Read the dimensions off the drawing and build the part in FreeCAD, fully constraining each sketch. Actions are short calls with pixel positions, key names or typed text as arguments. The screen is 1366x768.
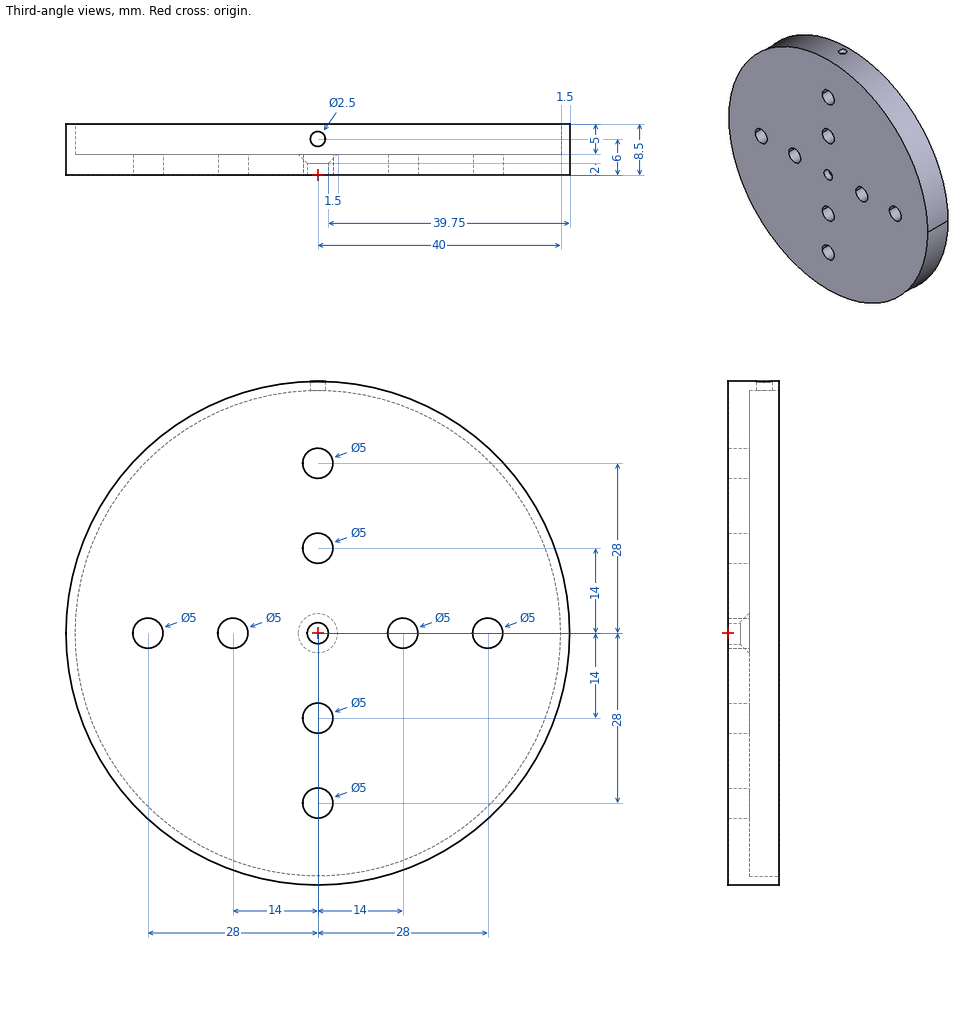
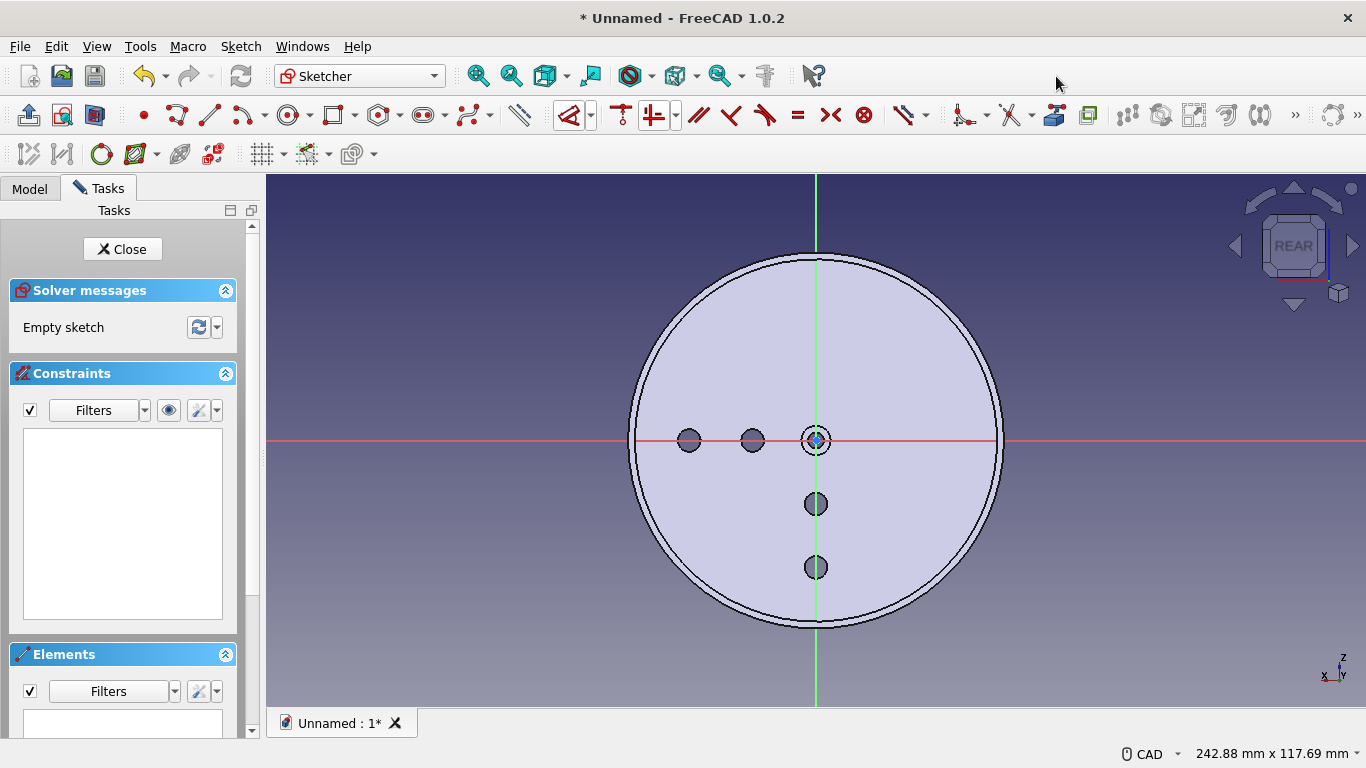
scroll(821, 372, up, 13)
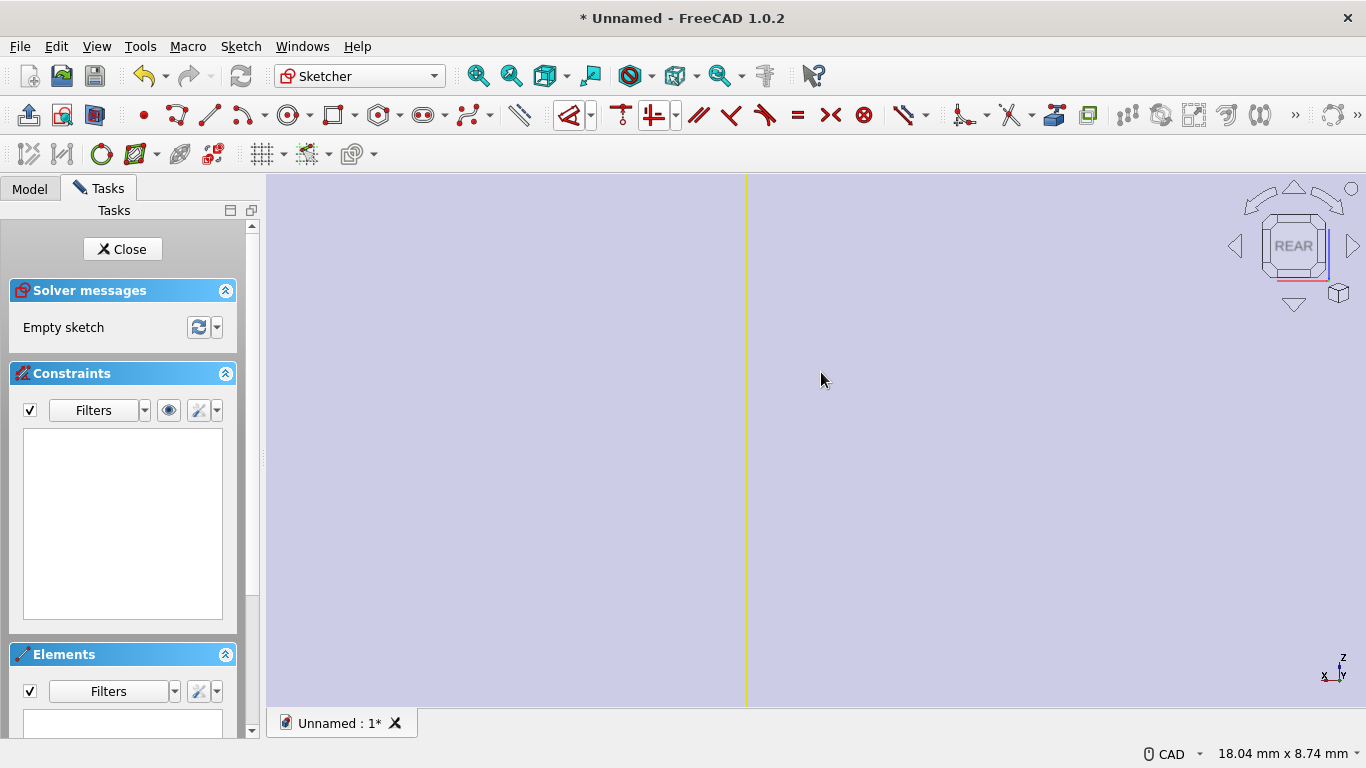
click(288, 116)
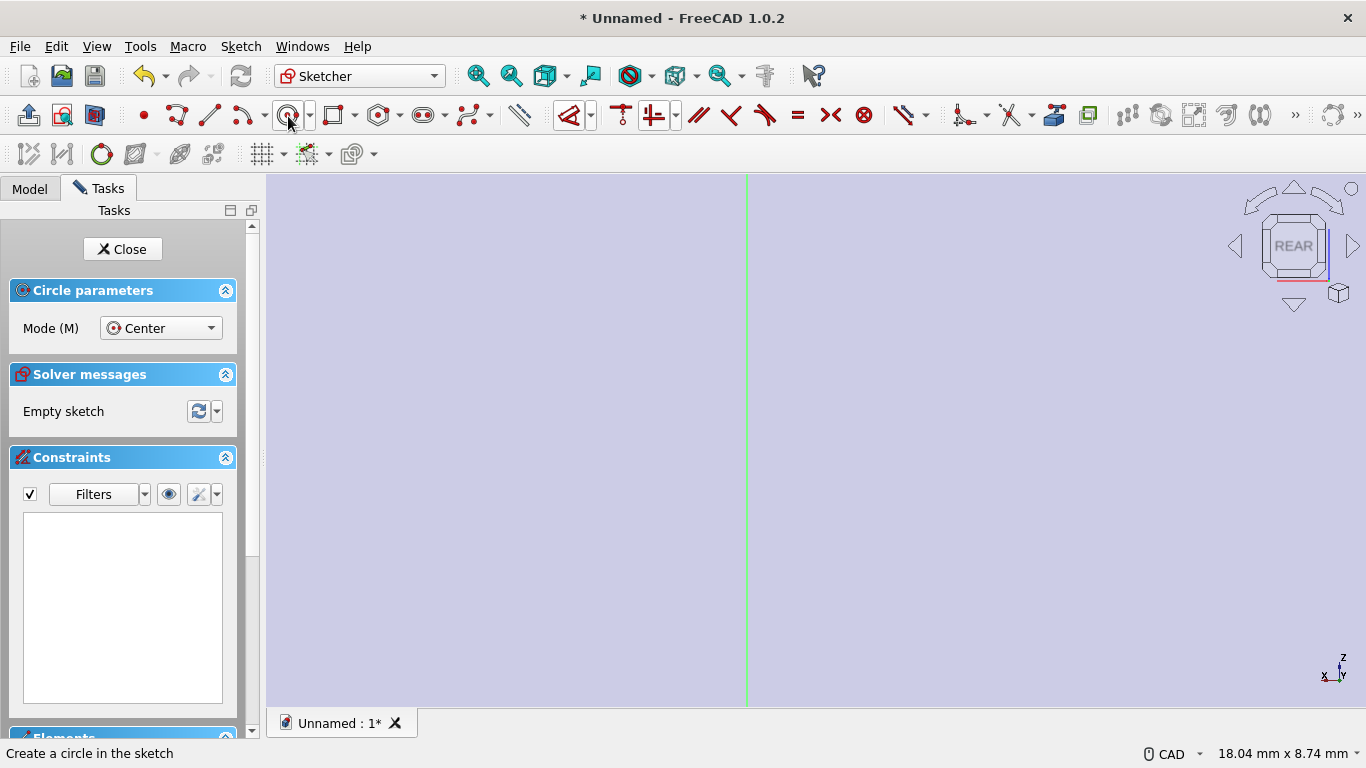
click(747, 436)
click(855, 328)
key(Escape)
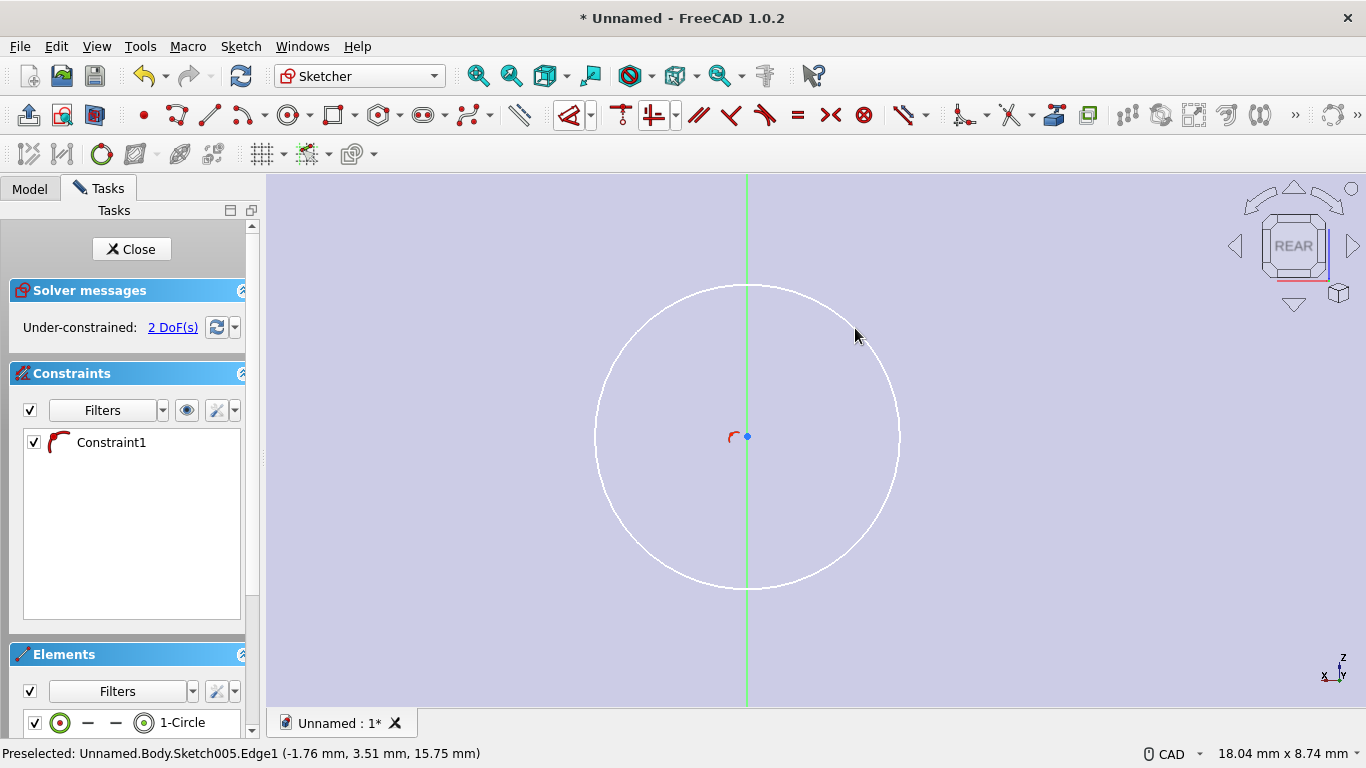
click(855, 329)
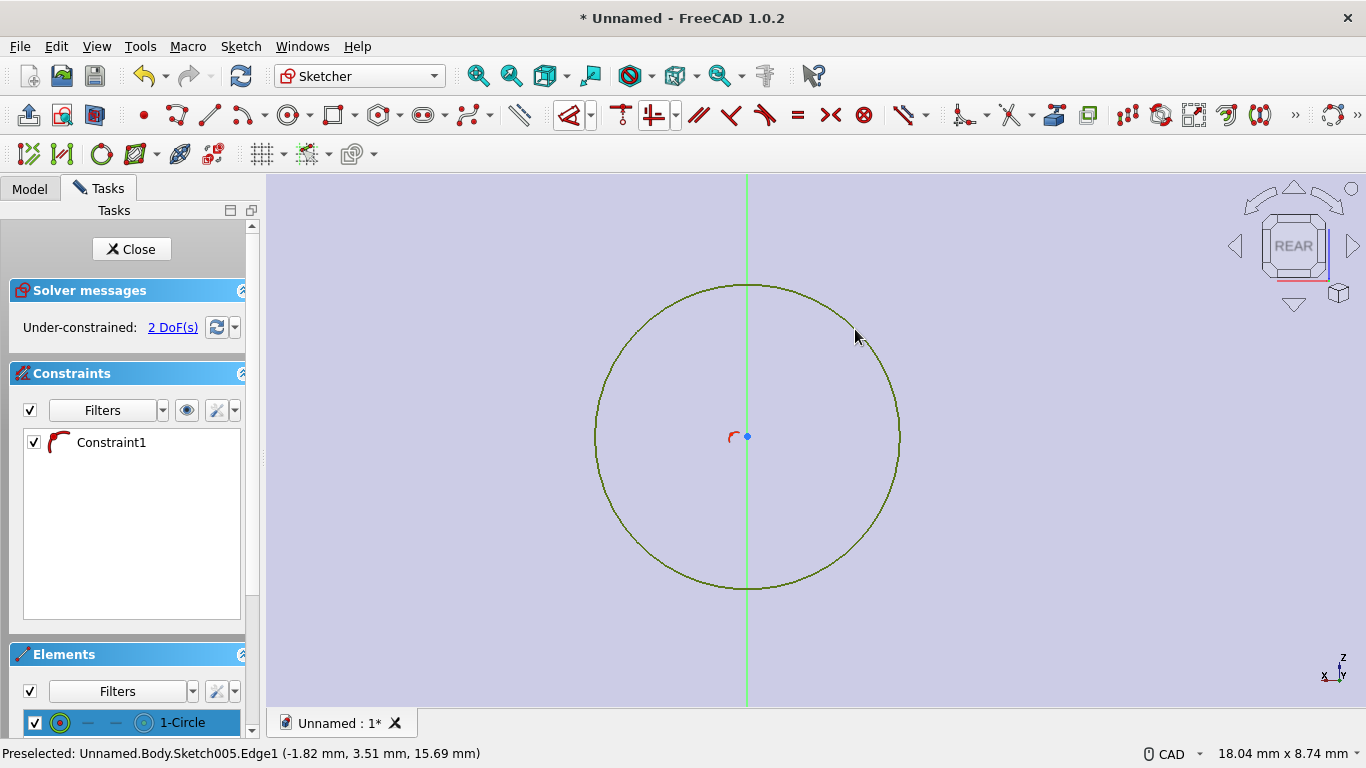
click(590, 116)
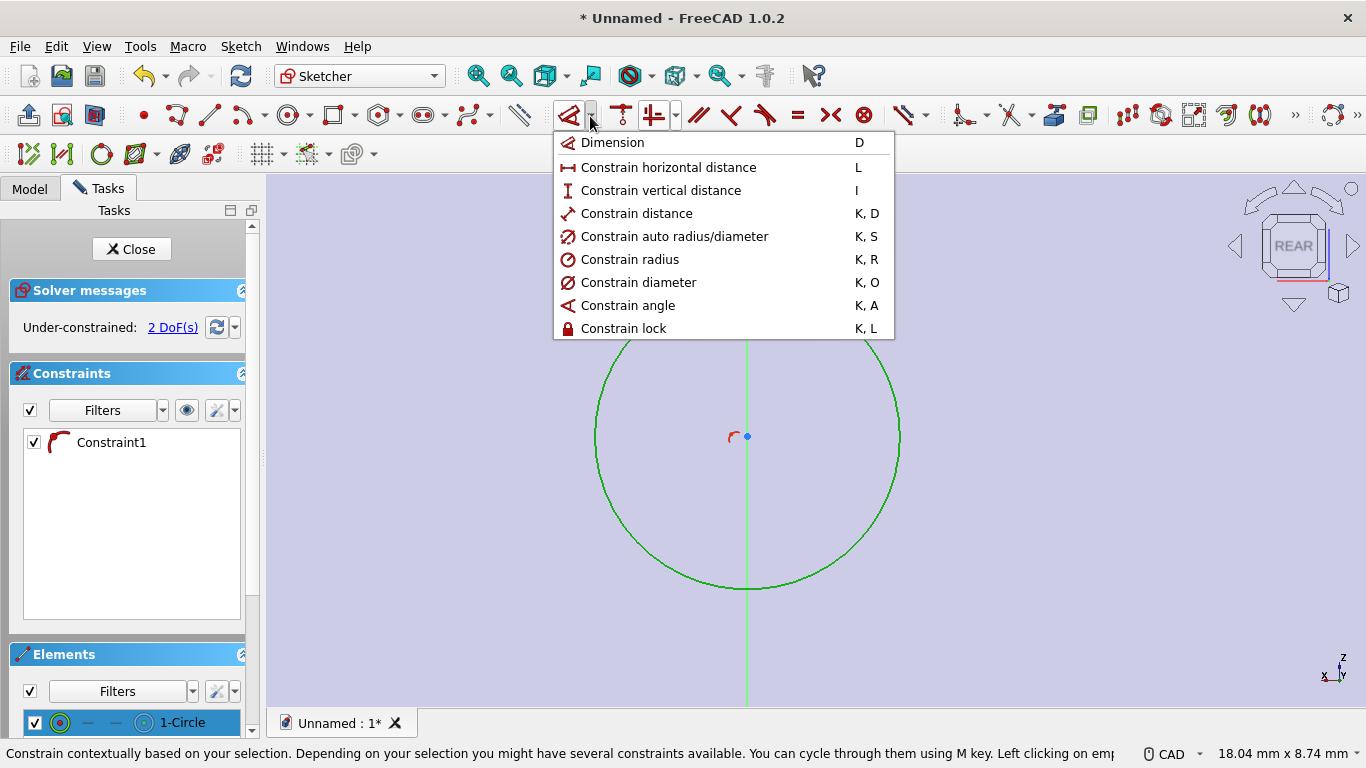
click(724, 282)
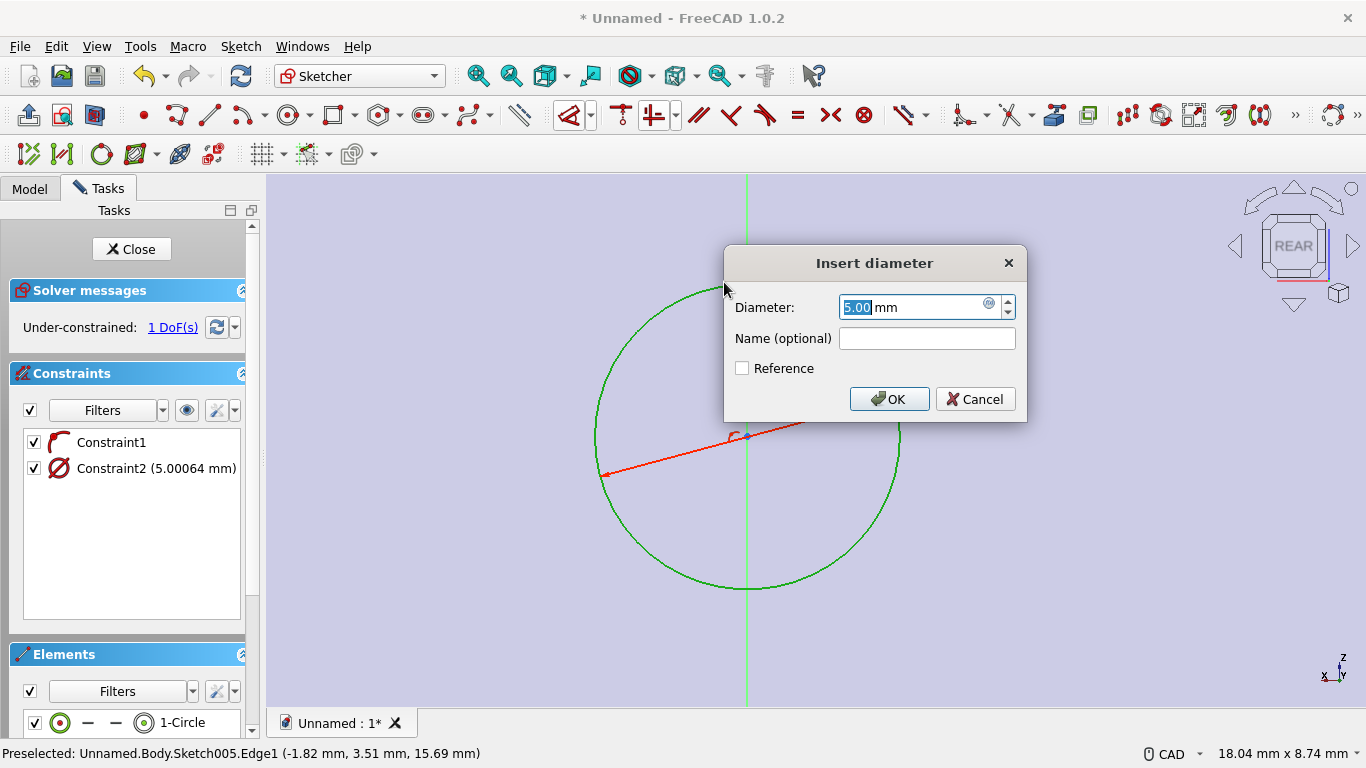
text(5)
key(Return)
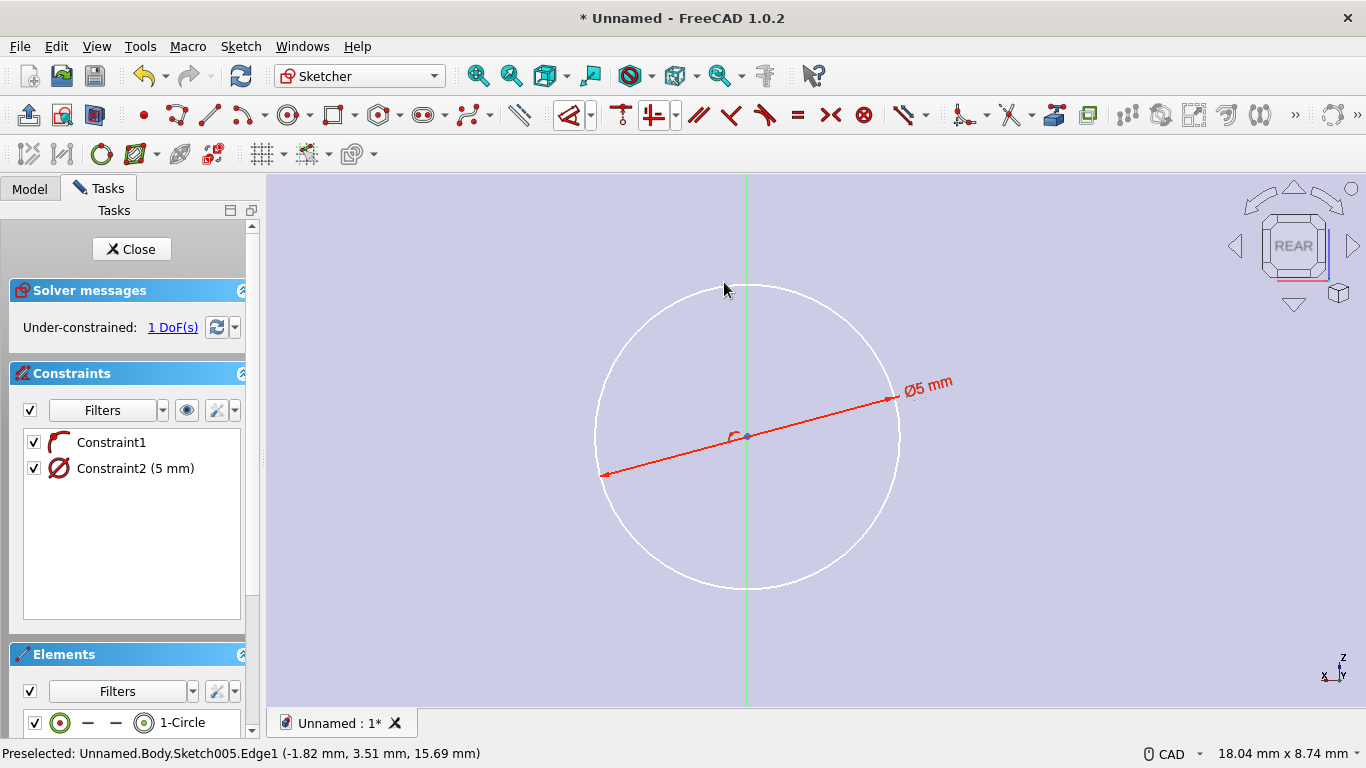
click(747, 437)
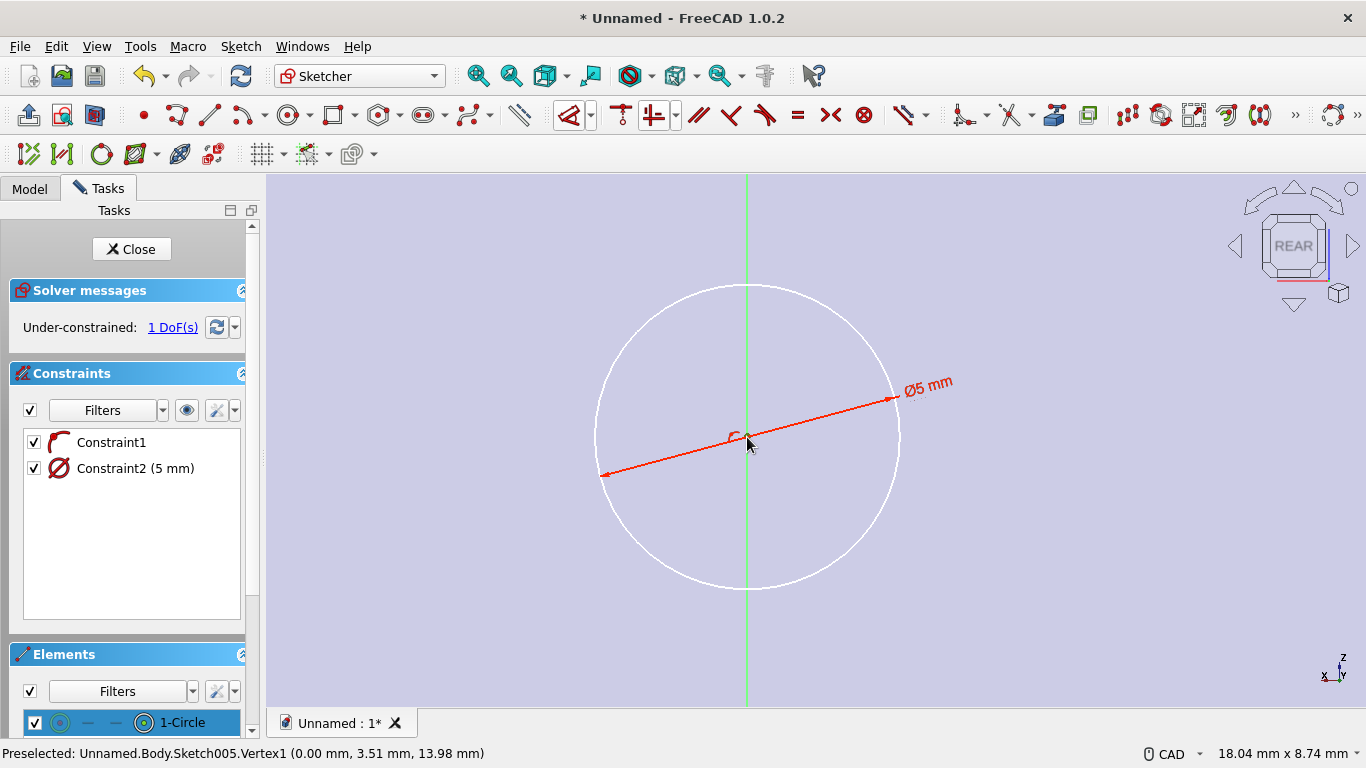
key(i)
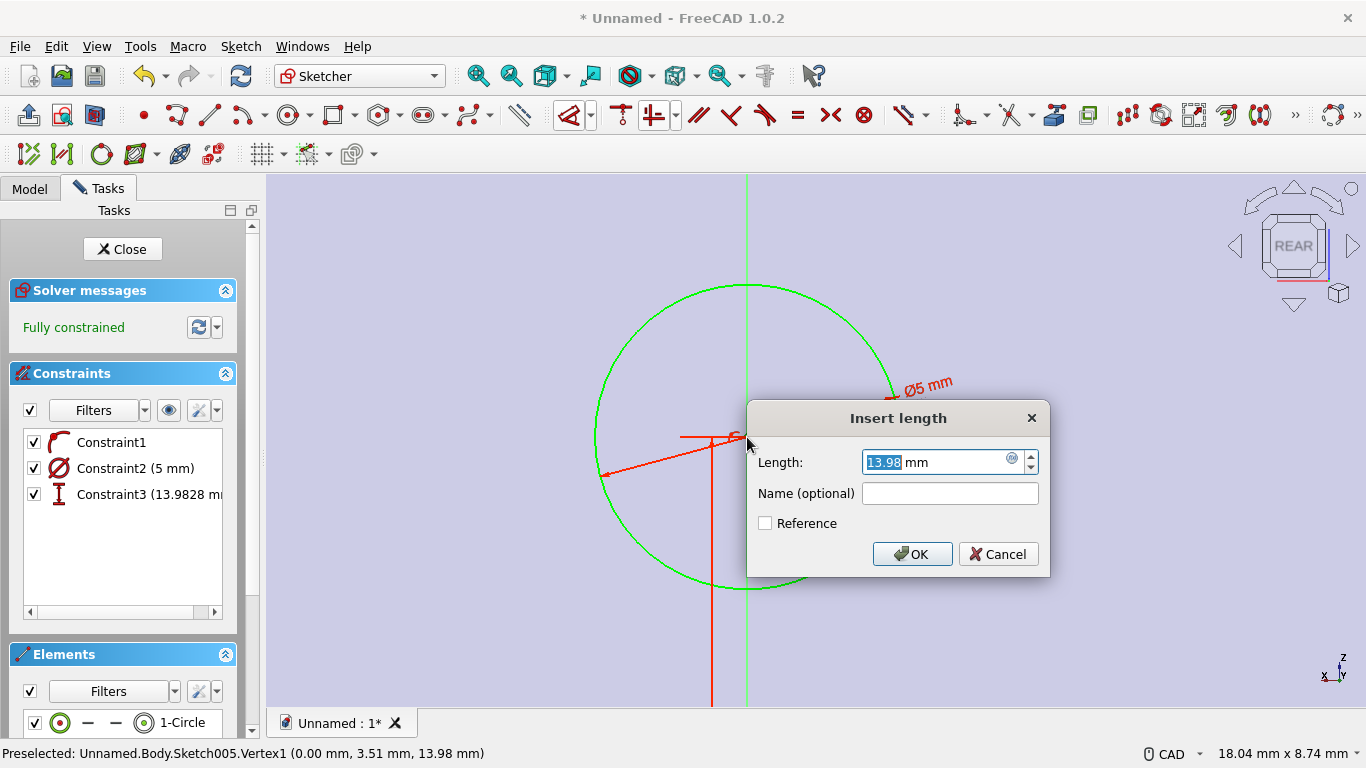
text(14)
key(Return)